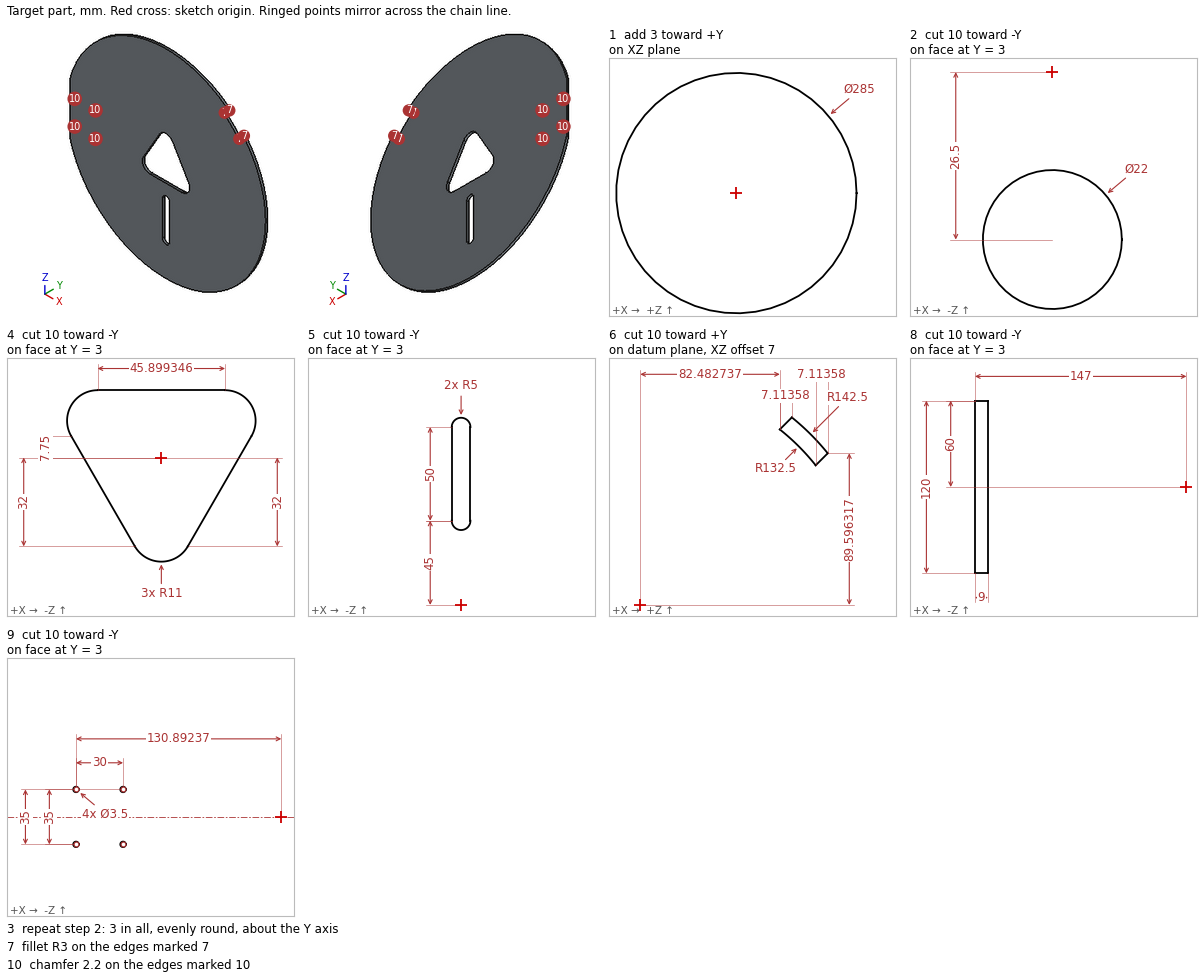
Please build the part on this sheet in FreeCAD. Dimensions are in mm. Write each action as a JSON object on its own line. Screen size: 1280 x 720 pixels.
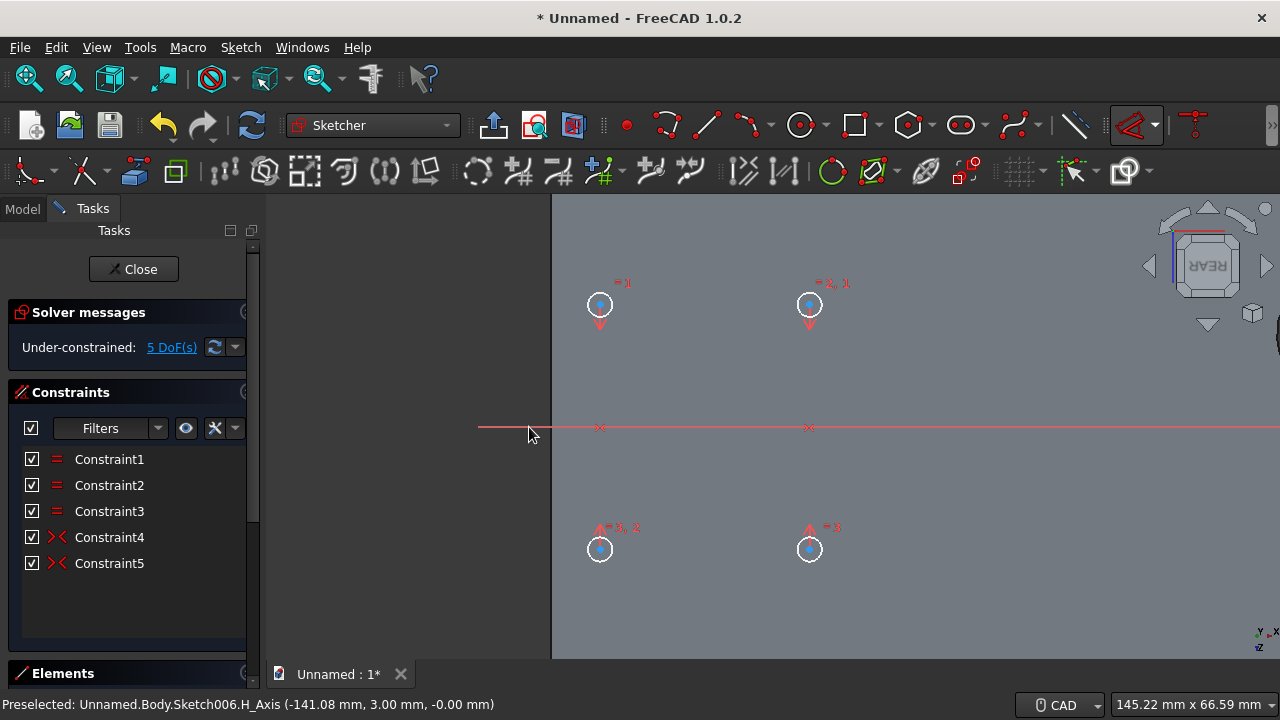
{"action": "scroll", "coordinate": [609, 296], "scroll_direction": "up", "scroll_amount": 3}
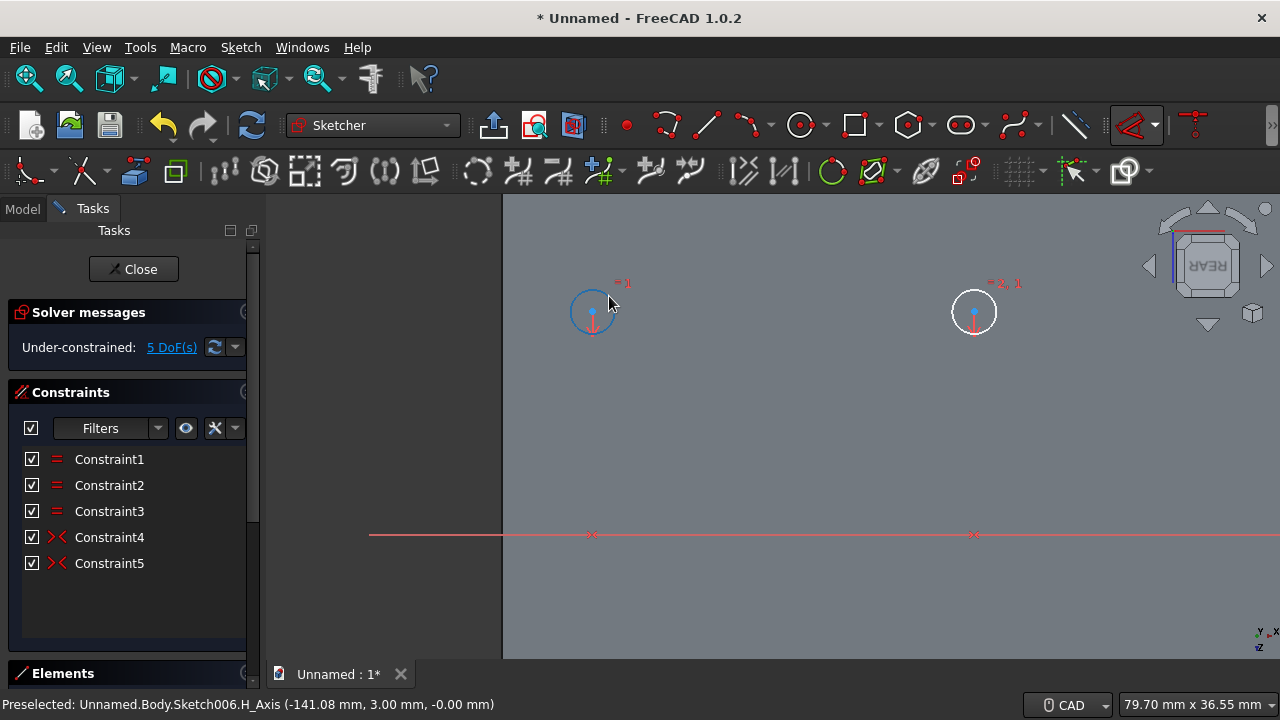
{"action": "left_click", "coordinate": [608, 296]}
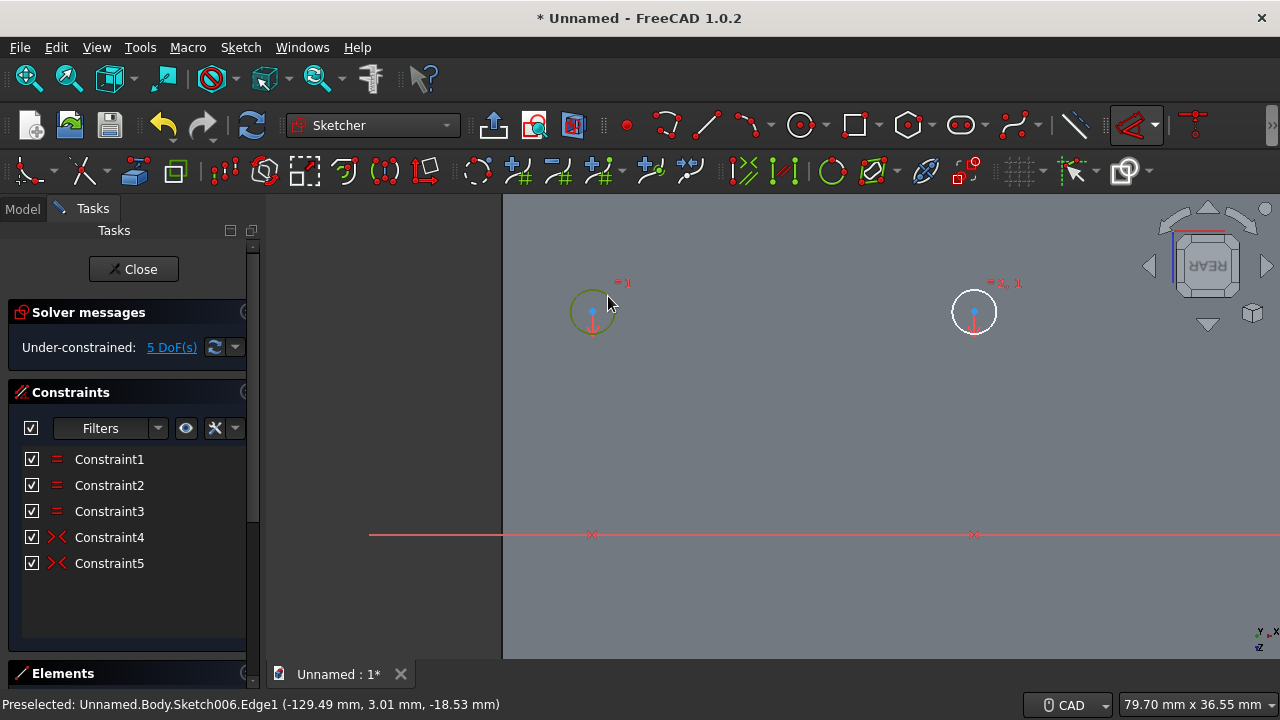
{"action": "left_click", "coordinate": [1158, 126]}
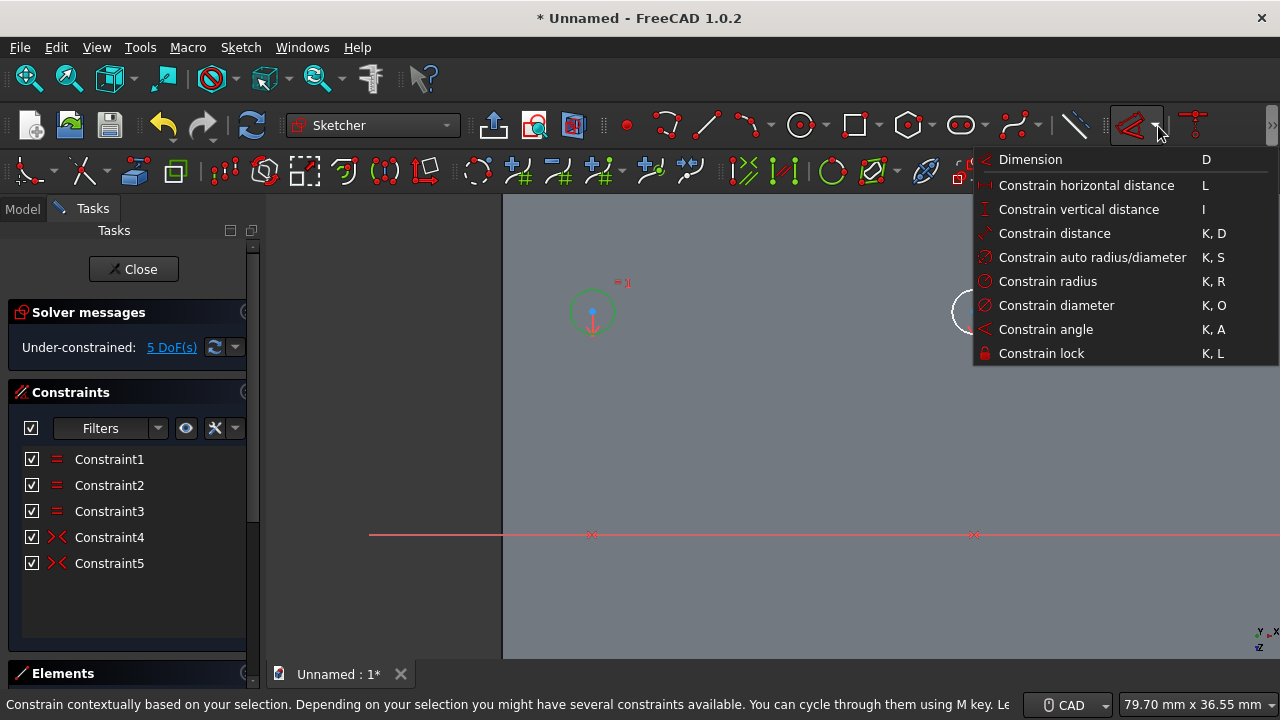
{"action": "left_click", "coordinate": [1126, 305]}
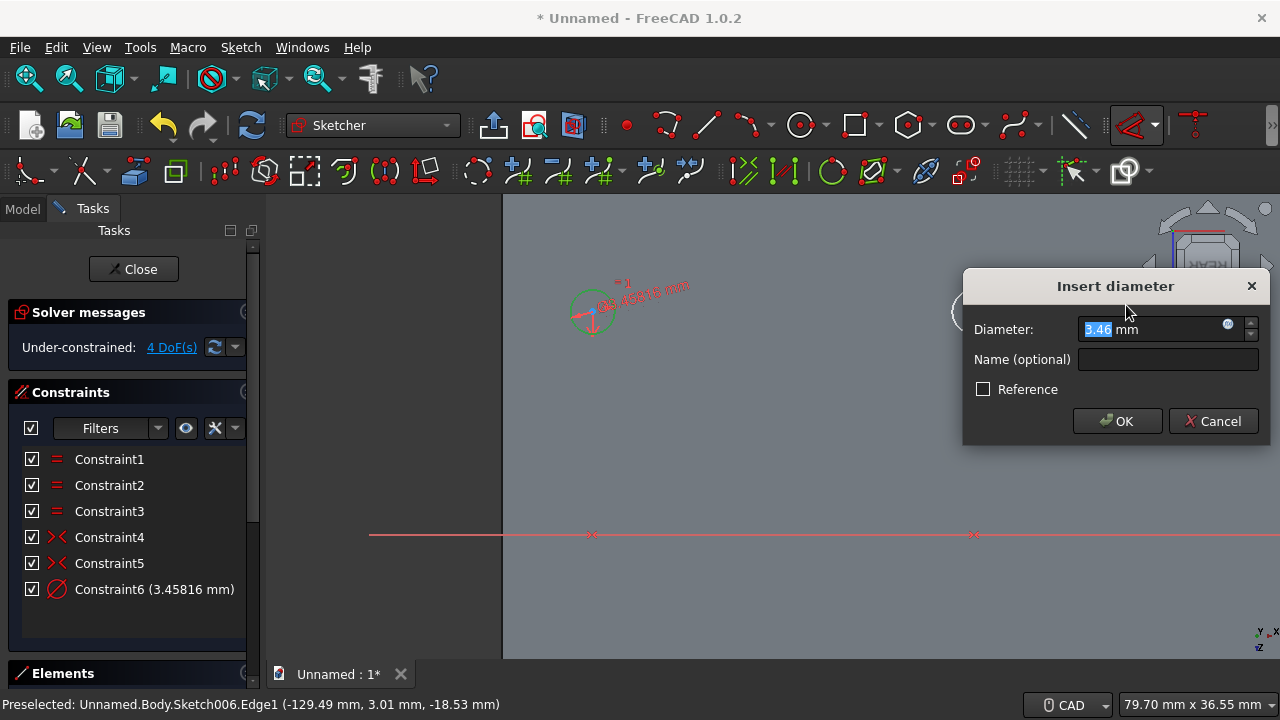
{"action": "type", "text": "3.5"}
{"action": "key", "text": "Return"}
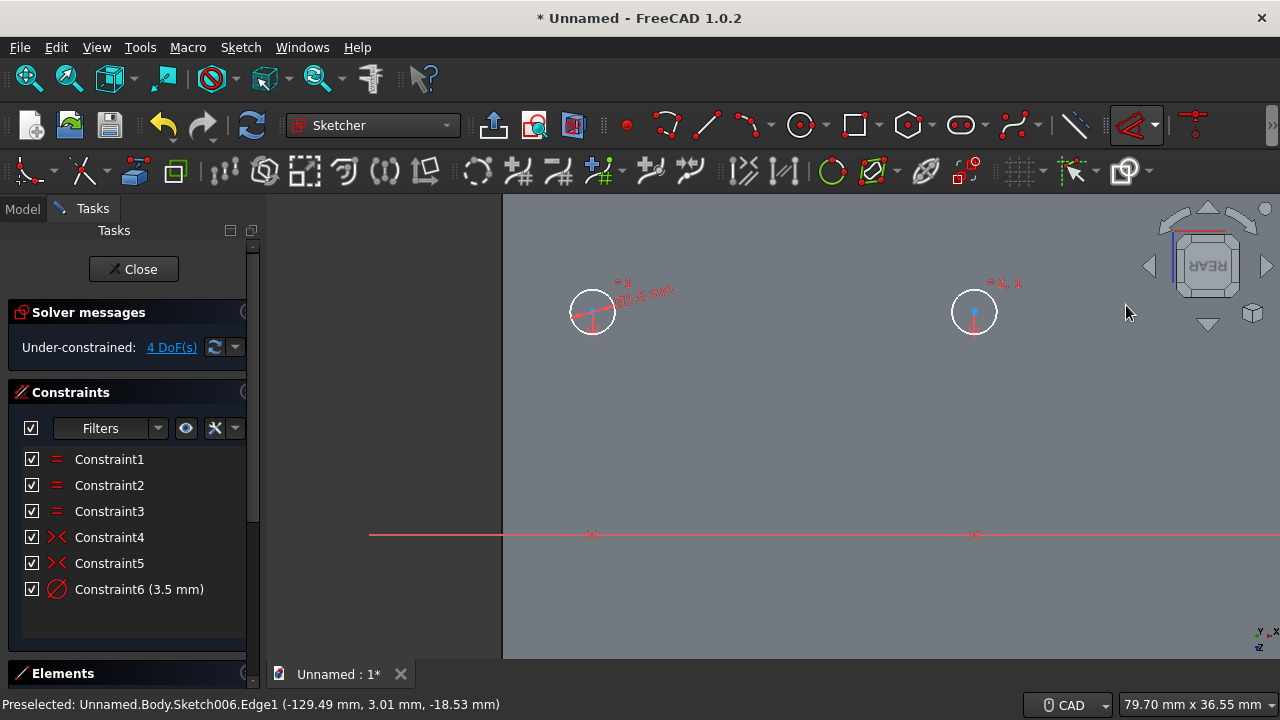
{"action": "left_click", "coordinate": [593, 312]}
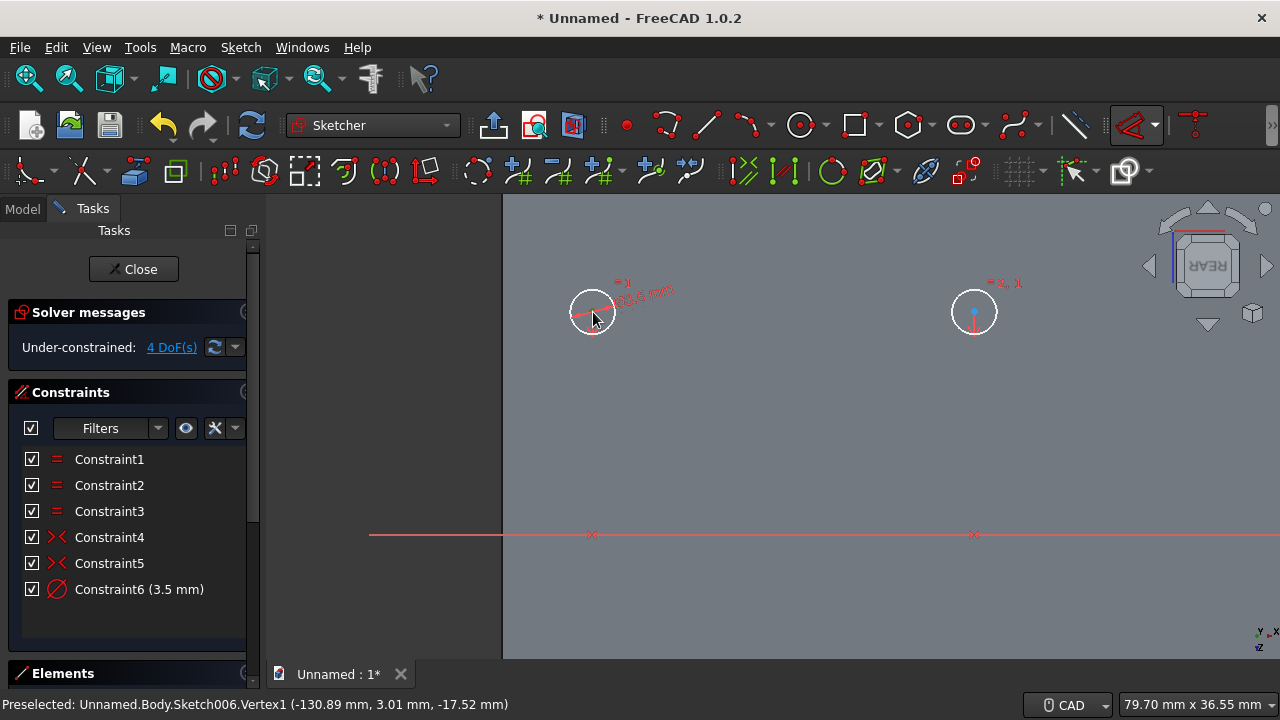
{"action": "left_click", "coordinate": [974, 312]}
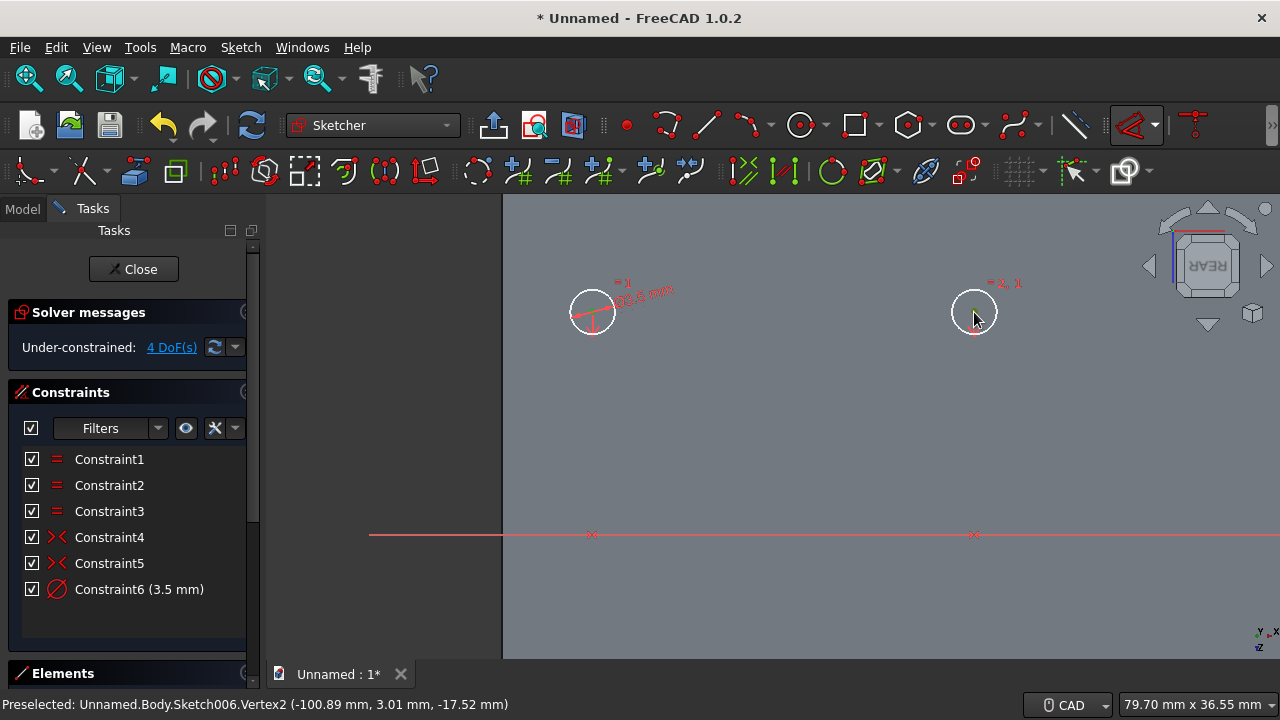
{"action": "key", "text": "l"}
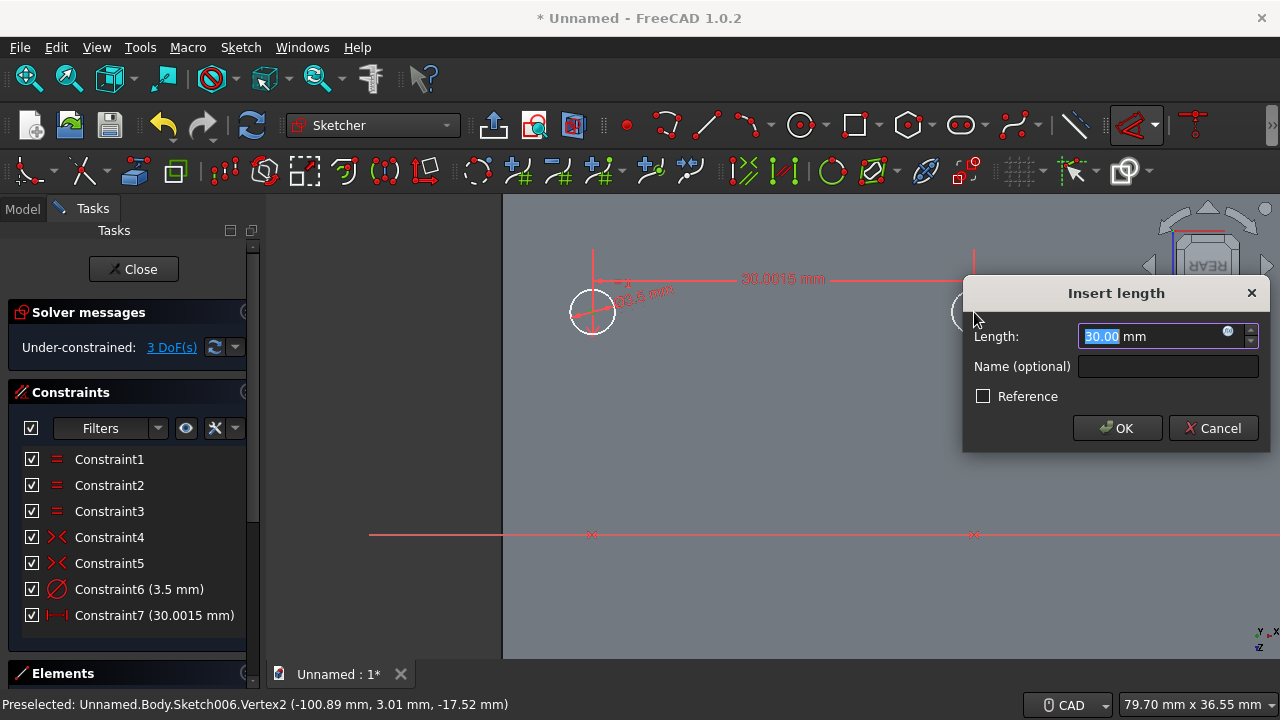
{"action": "type", "text": "30"}
{"action": "key", "text": "Return"}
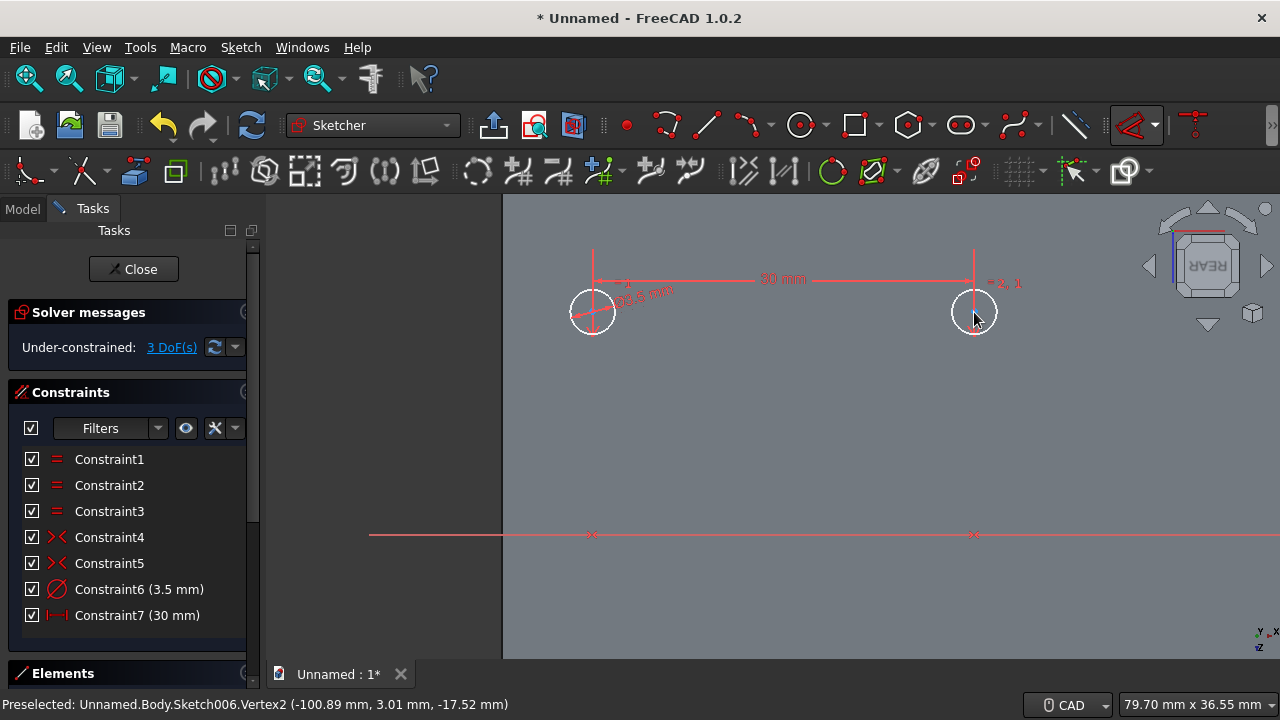
{"action": "left_click", "coordinate": [593, 312]}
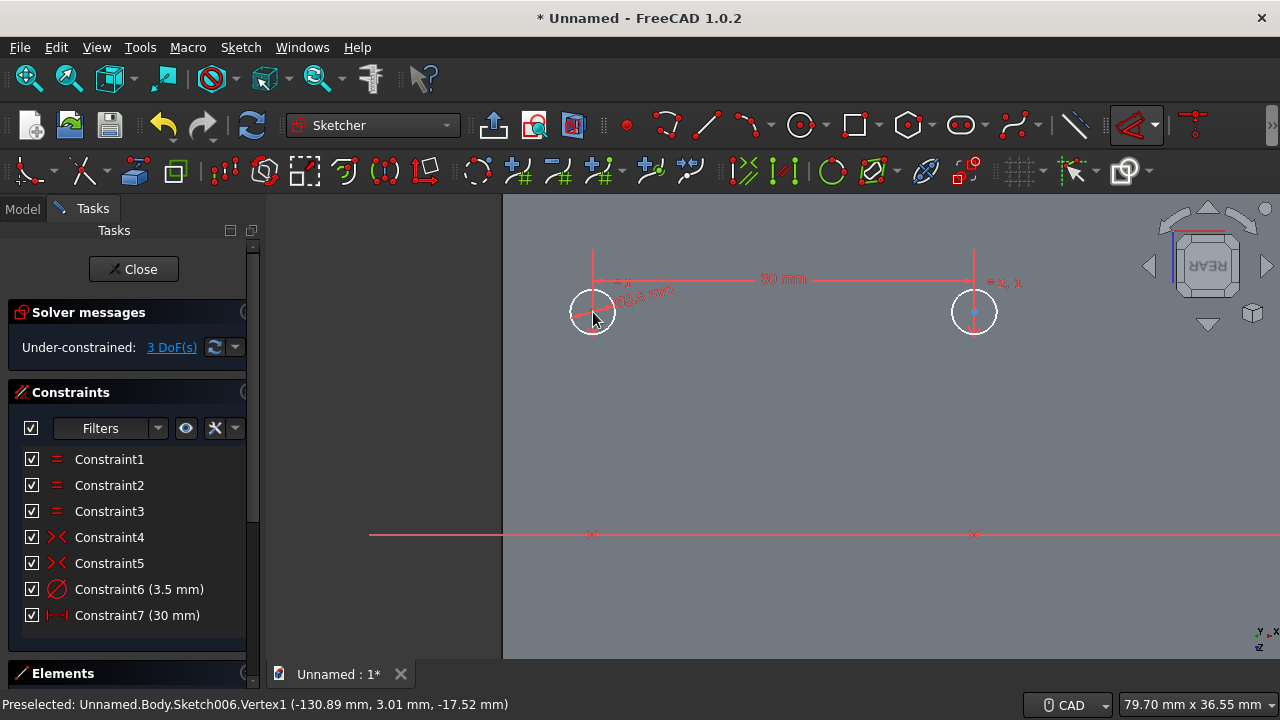
{"action": "scroll", "coordinate": [608, 295], "scroll_direction": "down", "scroll_amount": 3}